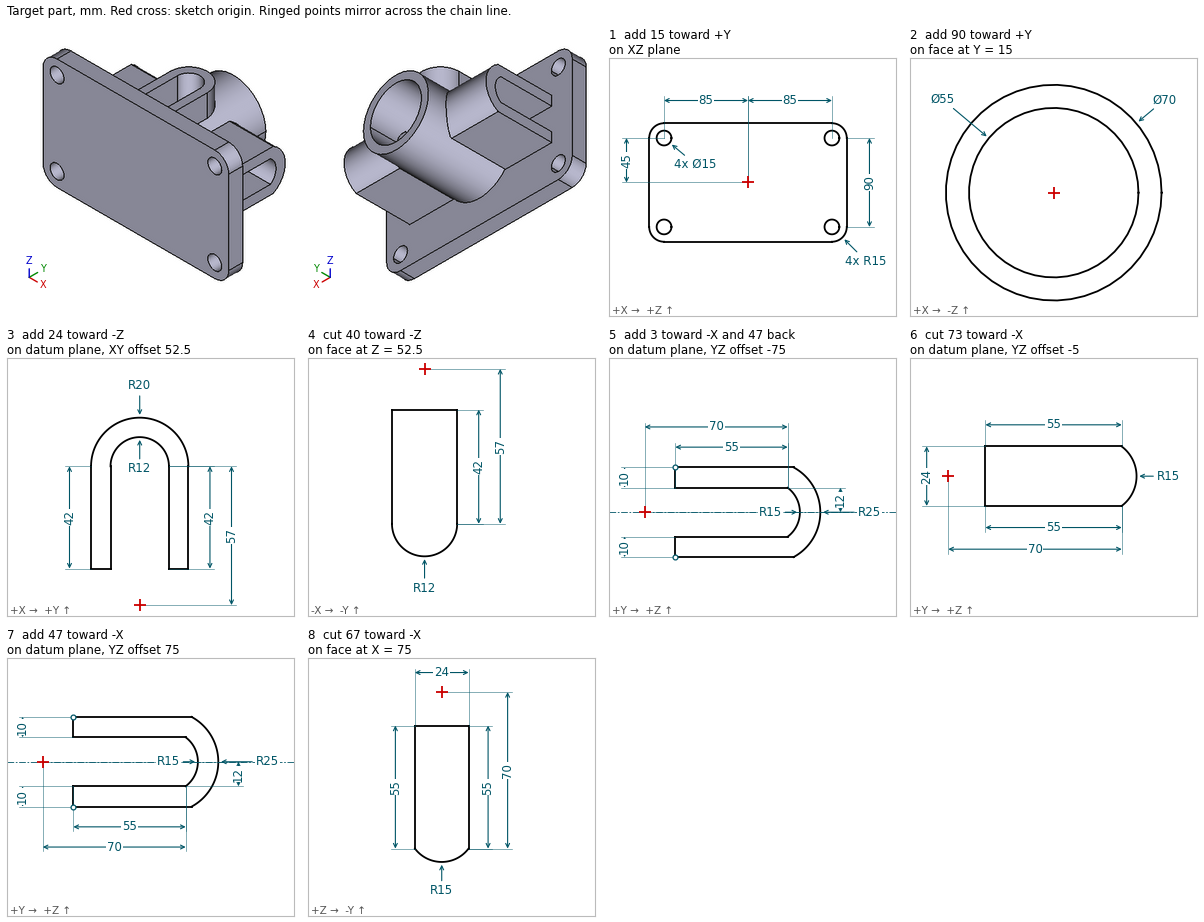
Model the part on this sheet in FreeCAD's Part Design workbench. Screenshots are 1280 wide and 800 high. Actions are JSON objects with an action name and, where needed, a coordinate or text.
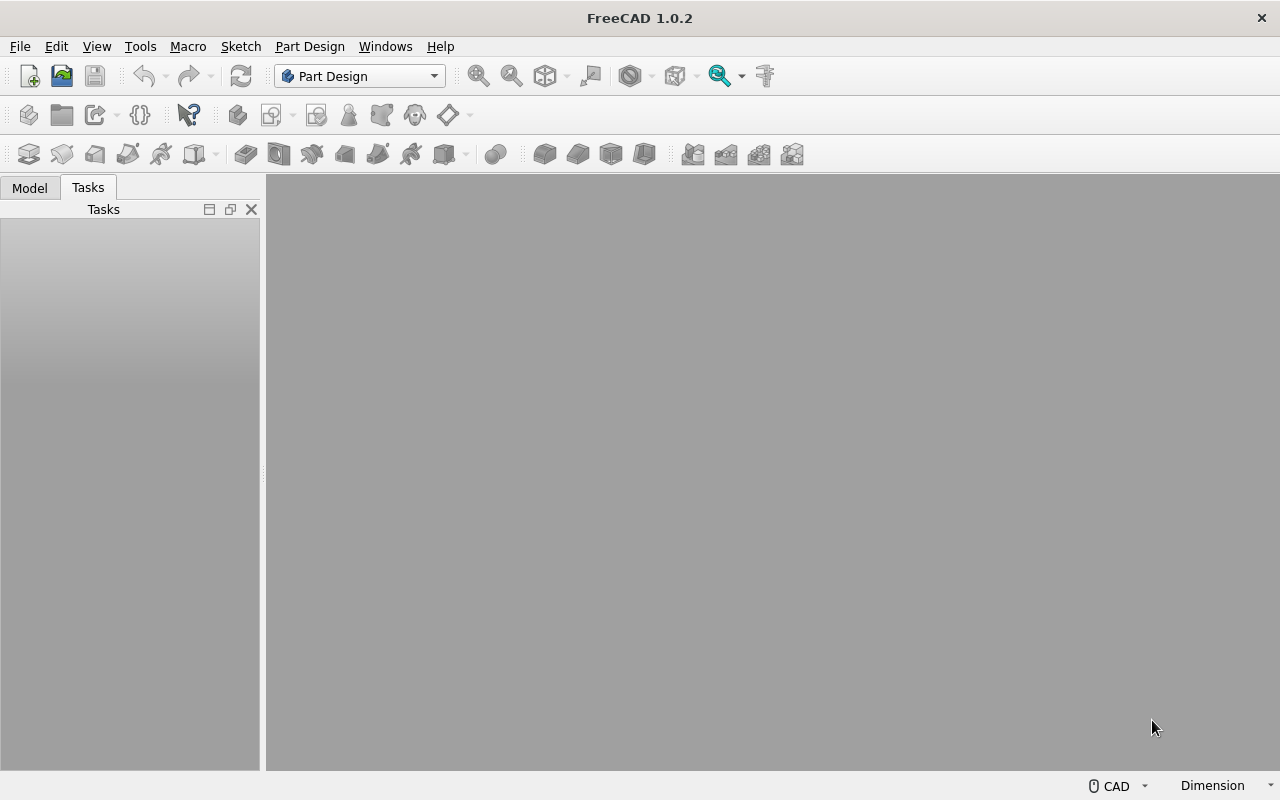
{"action": "left_click", "coordinate": [29, 76]}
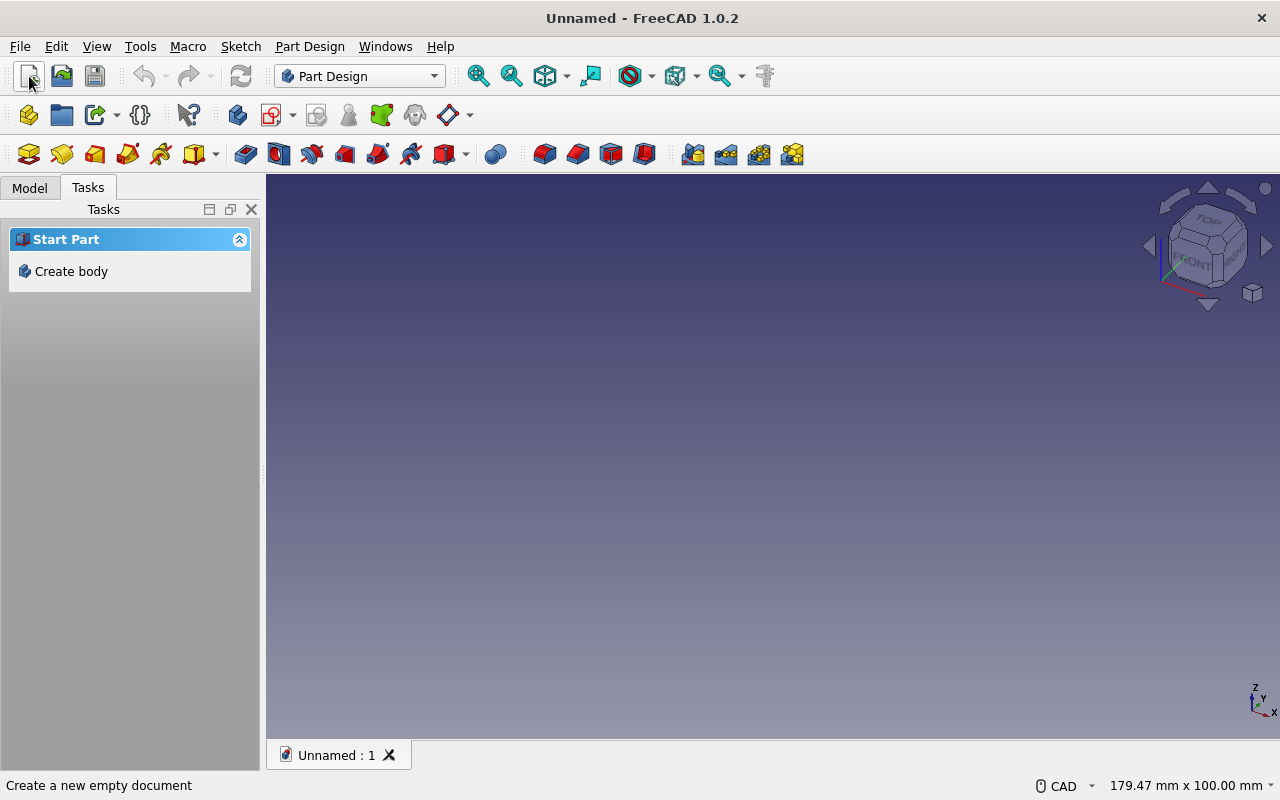
{"action": "left_click", "coordinate": [270, 116]}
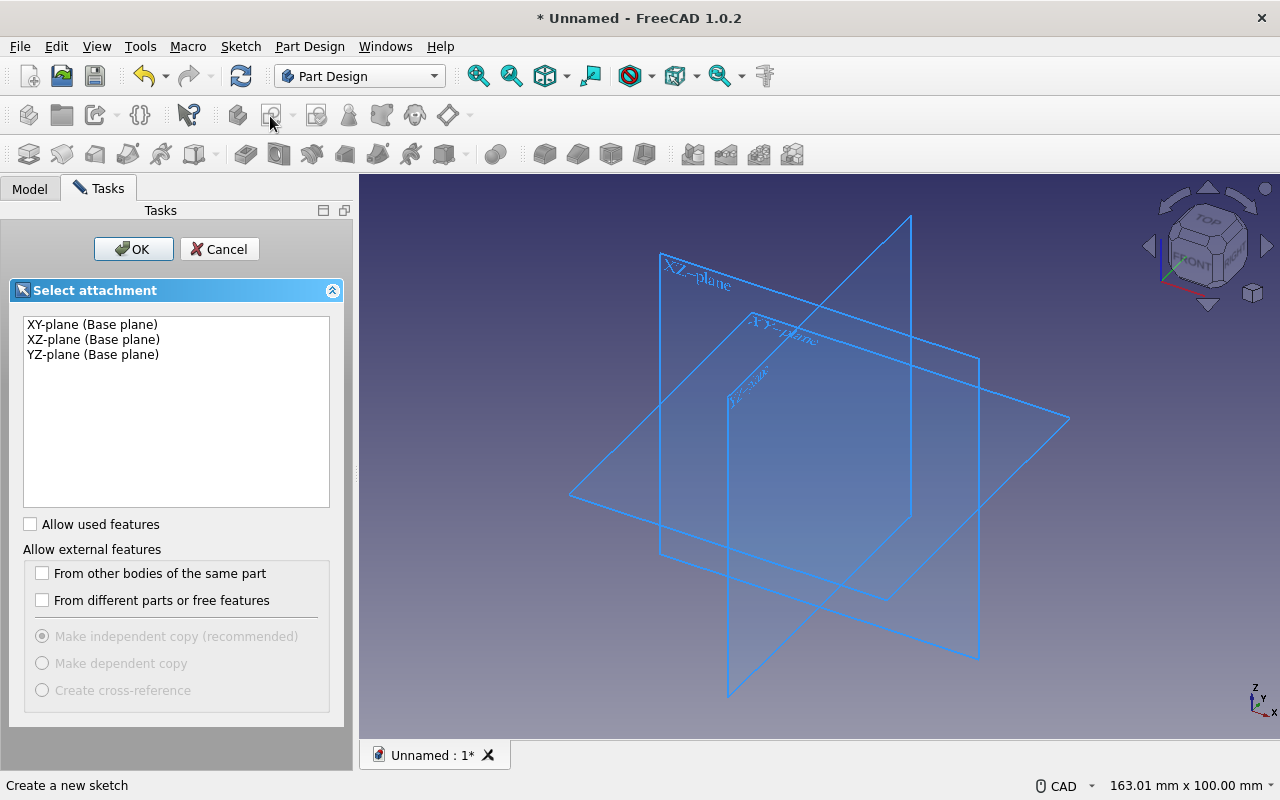
{"action": "left_click", "coordinate": [84, 340]}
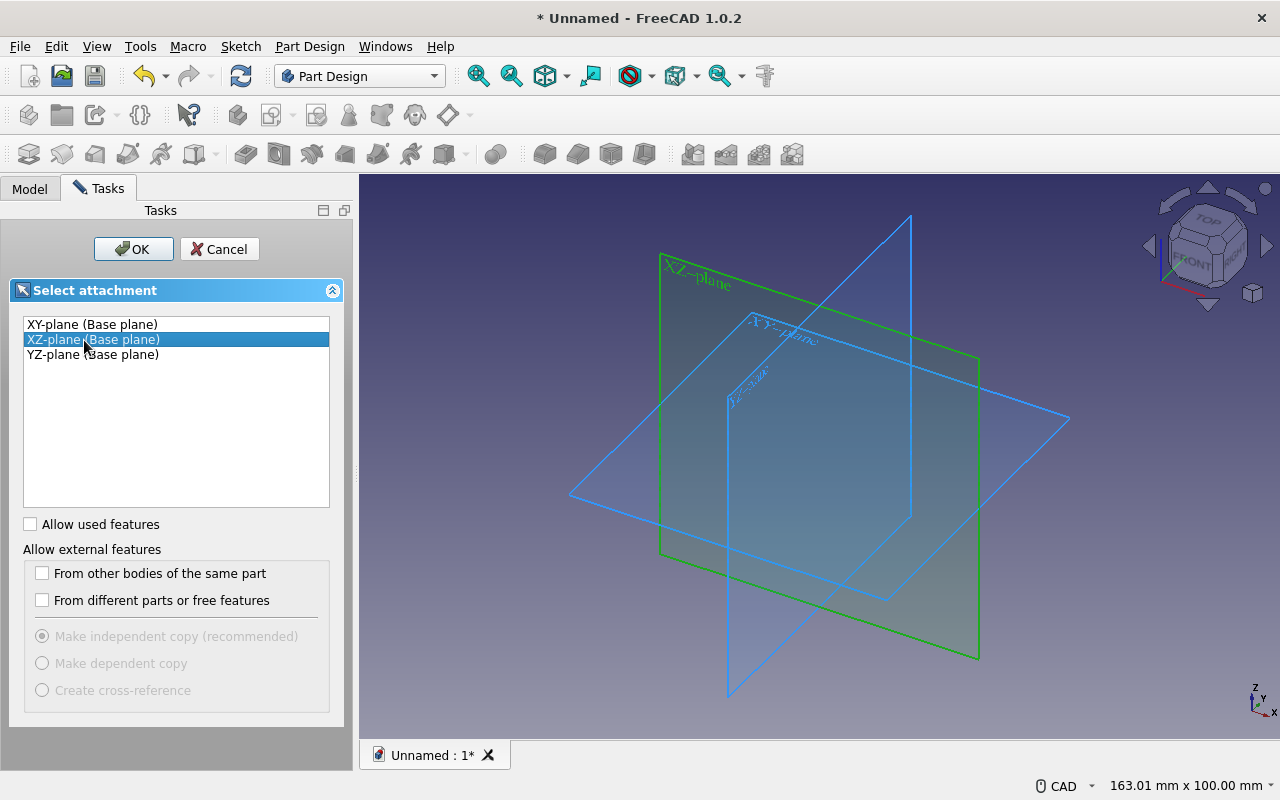
{"action": "left_click", "coordinate": [134, 249]}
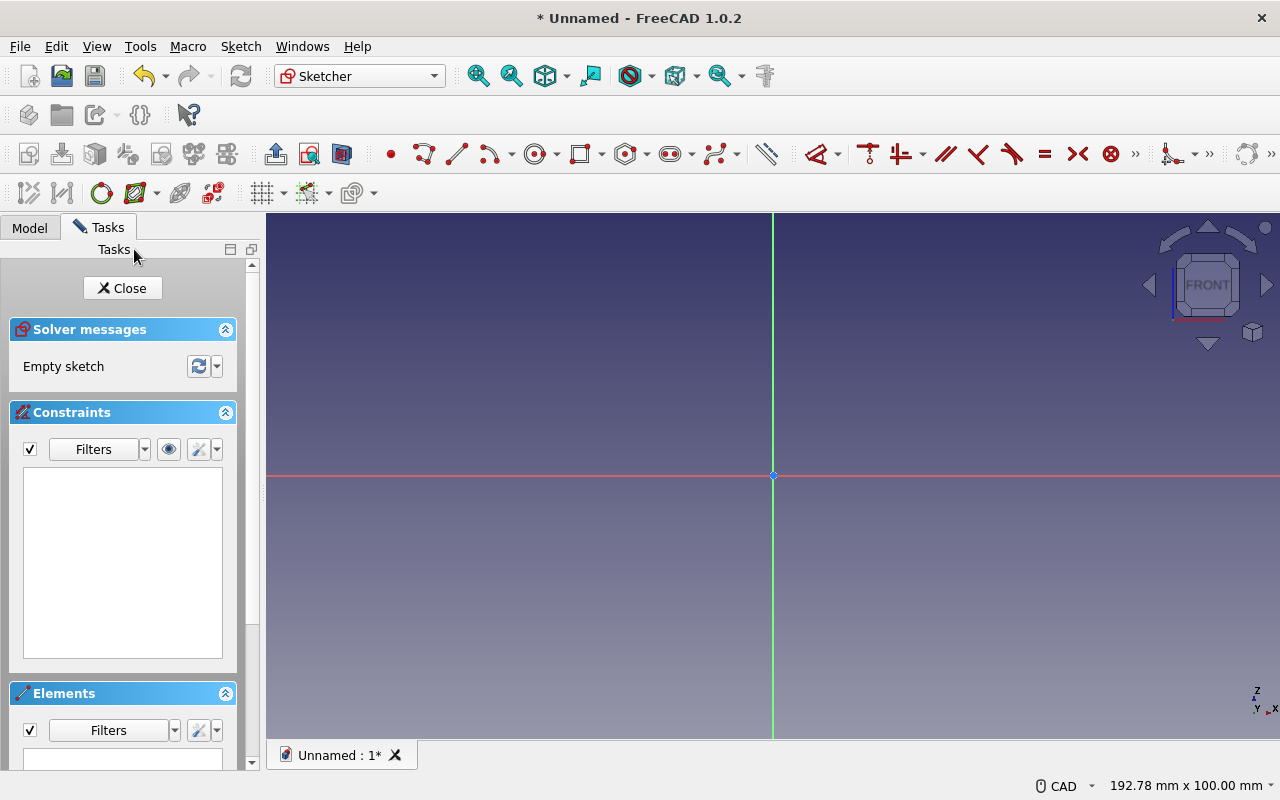
{"action": "scroll", "coordinate": [621, 476], "scroll_direction": "down", "scroll_amount": 3}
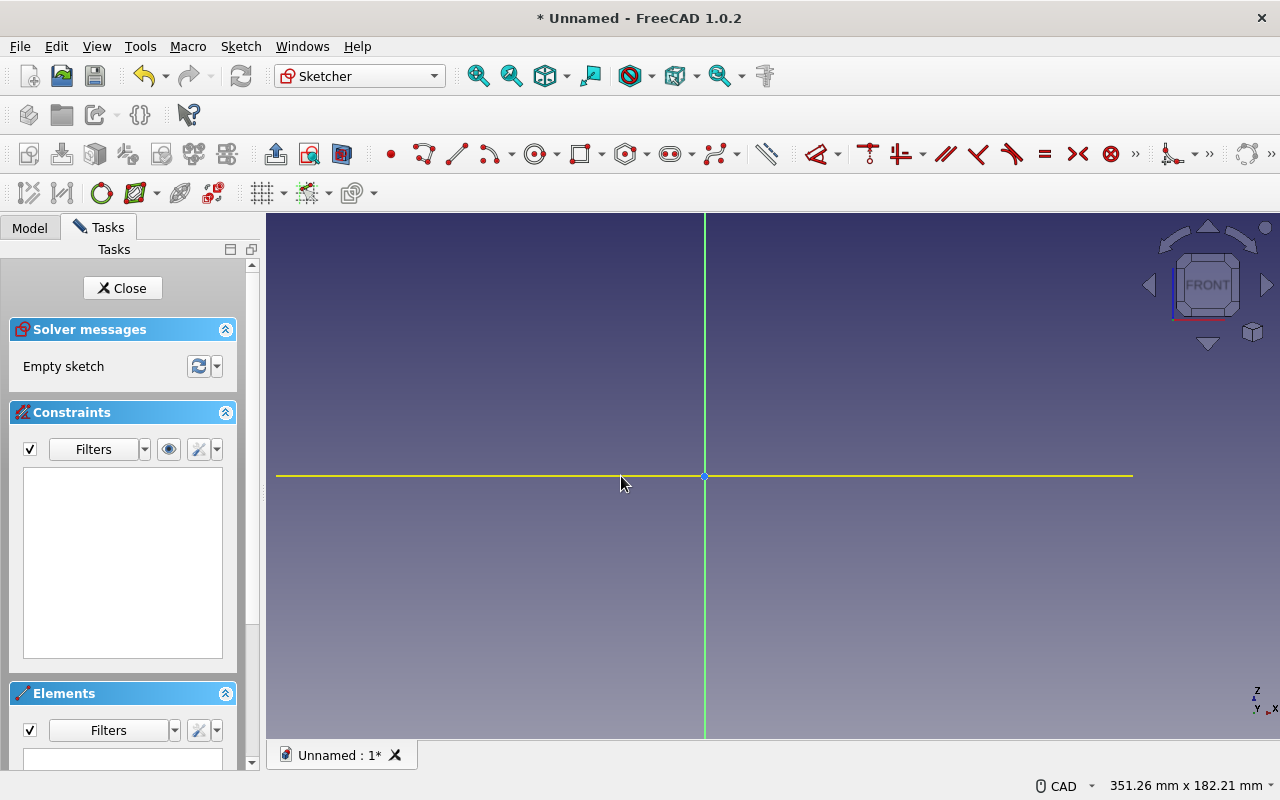
{"action": "key", "text": "g l"}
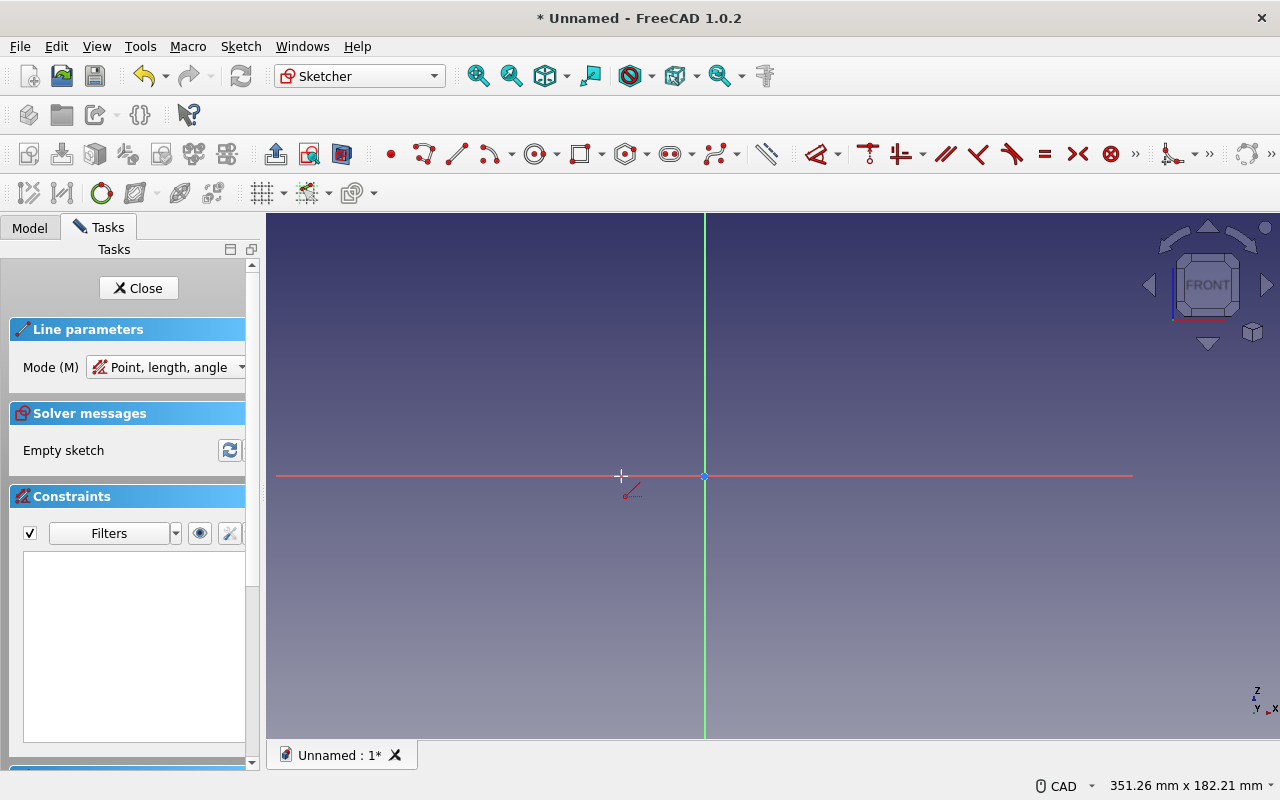
{"action": "left_click", "coordinate": [459, 303]}
{"action": "left_click", "coordinate": [950, 303]}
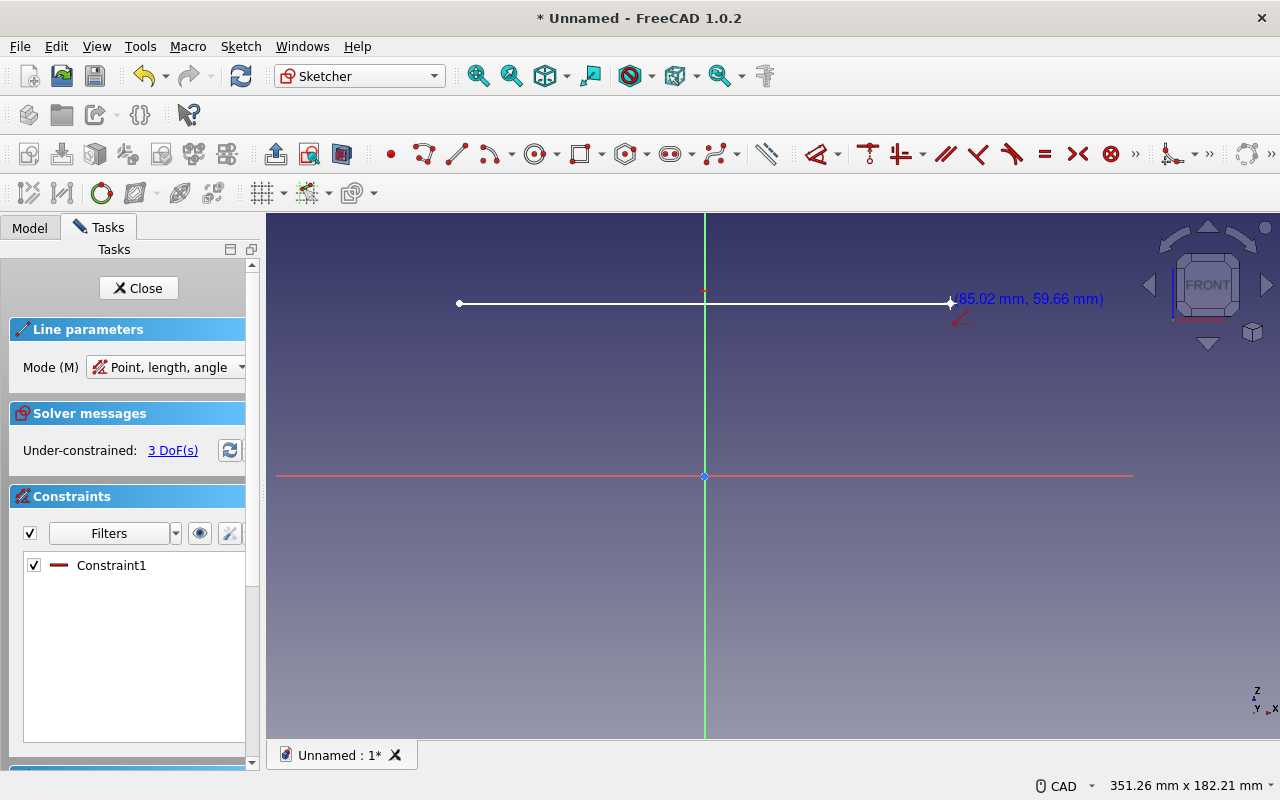
{"action": "left_click", "coordinate": [993, 346]}
{"action": "left_click", "coordinate": [993, 606]}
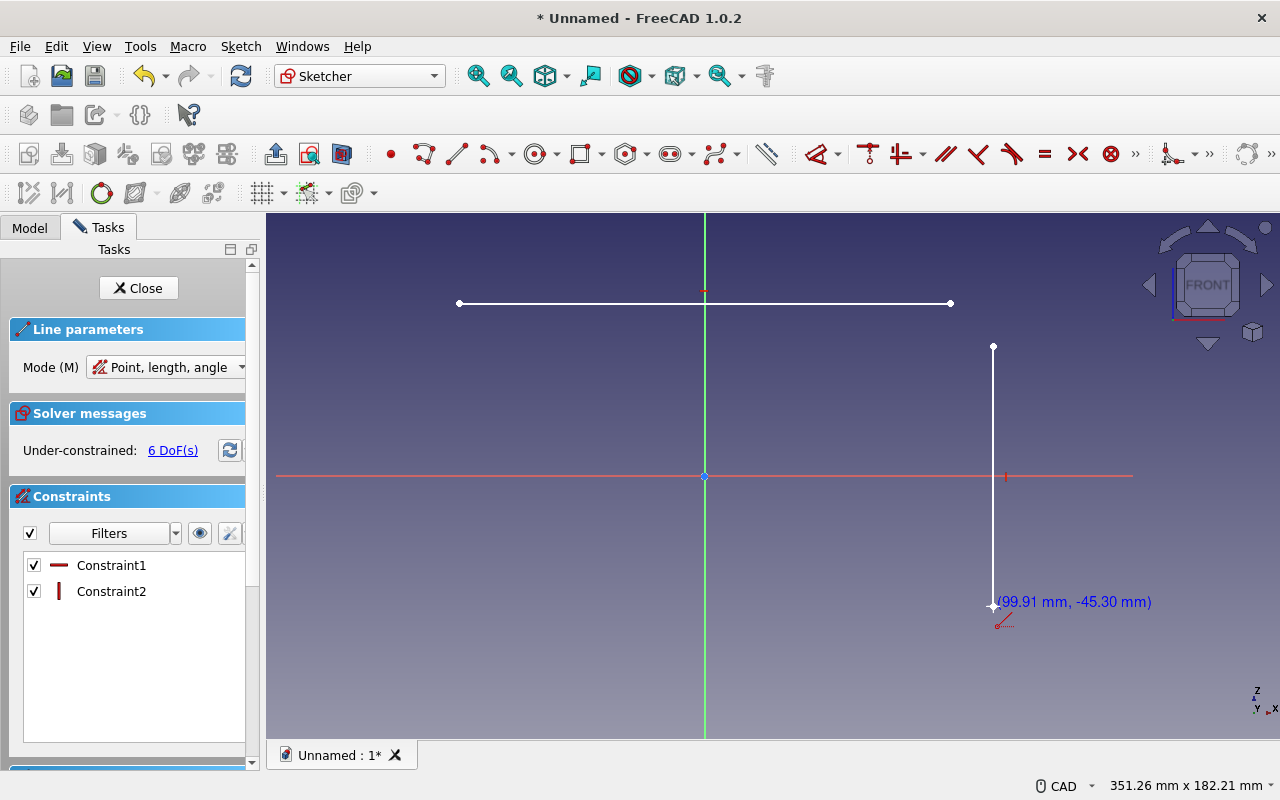
{"action": "left_click", "coordinate": [950, 649]}
{"action": "left_click", "coordinate": [459, 649]}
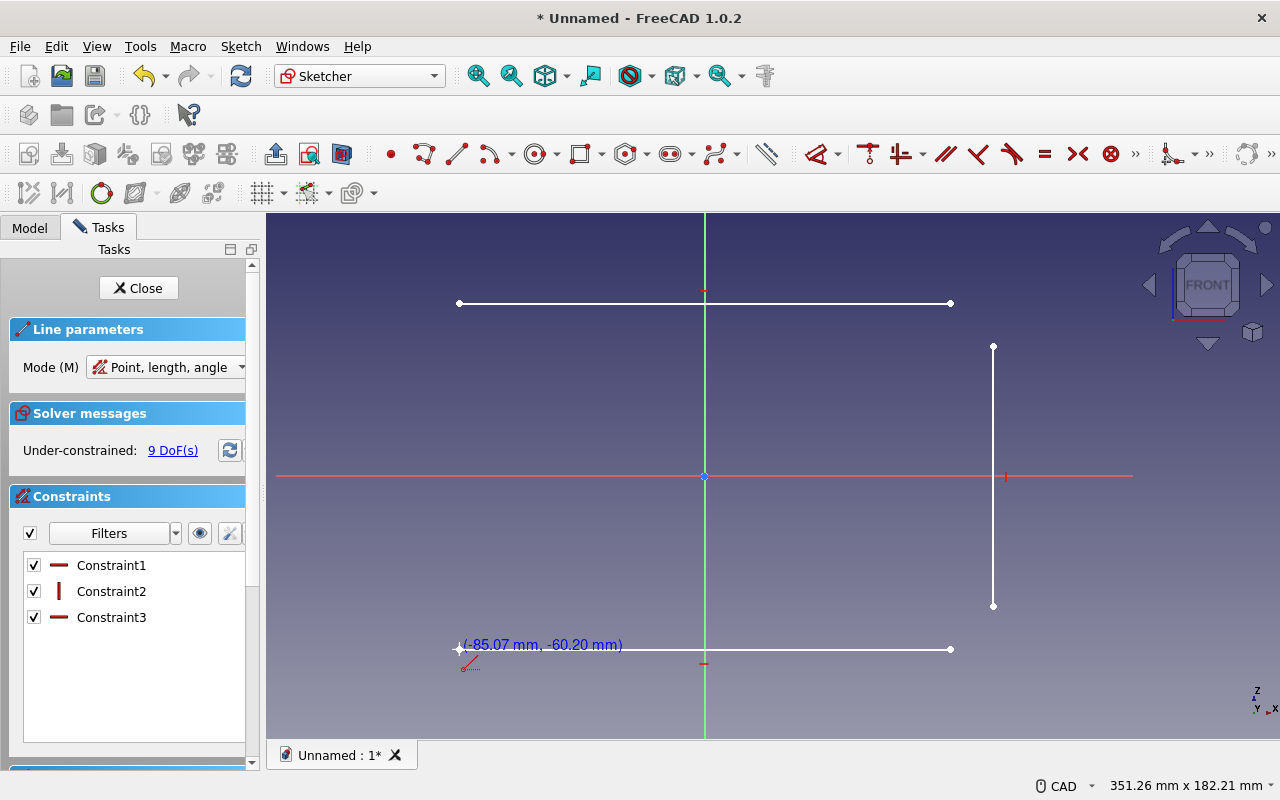
{"action": "left_click", "coordinate": [416, 606]}
{"action": "left_click", "coordinate": [416, 346]}